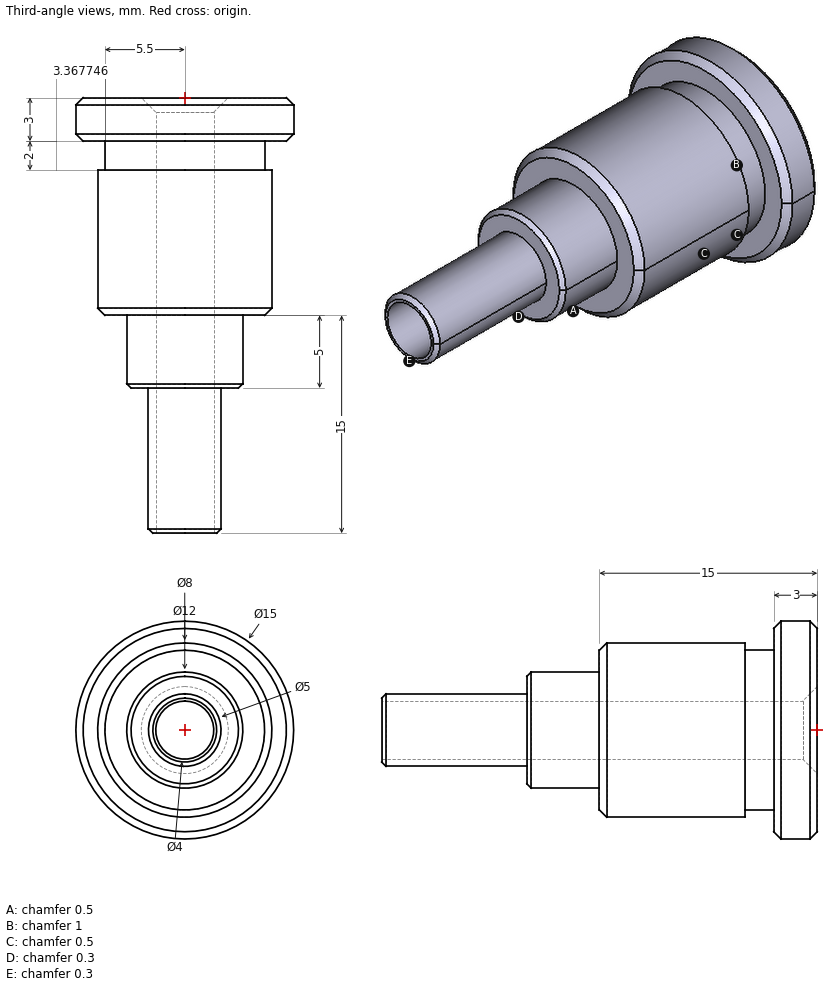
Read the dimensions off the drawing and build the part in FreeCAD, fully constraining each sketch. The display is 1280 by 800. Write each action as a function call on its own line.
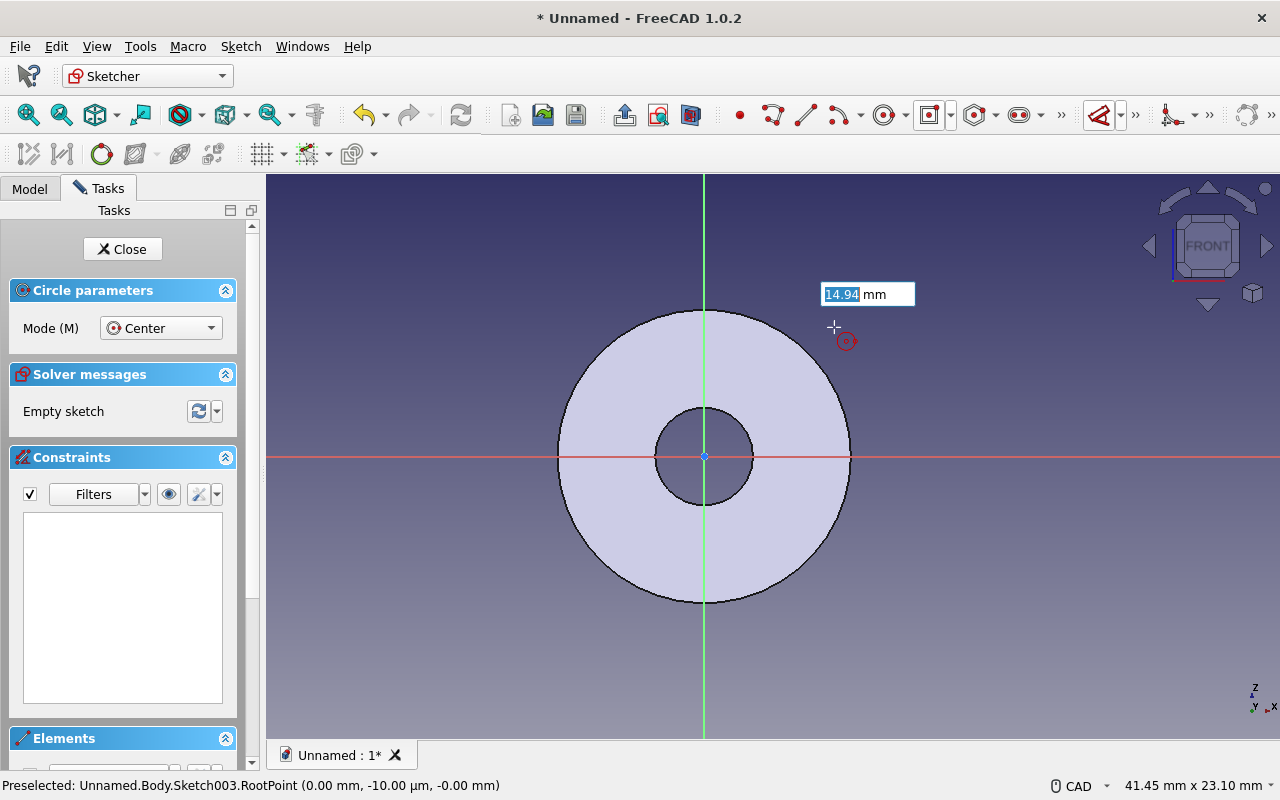
text(15)
key(Return)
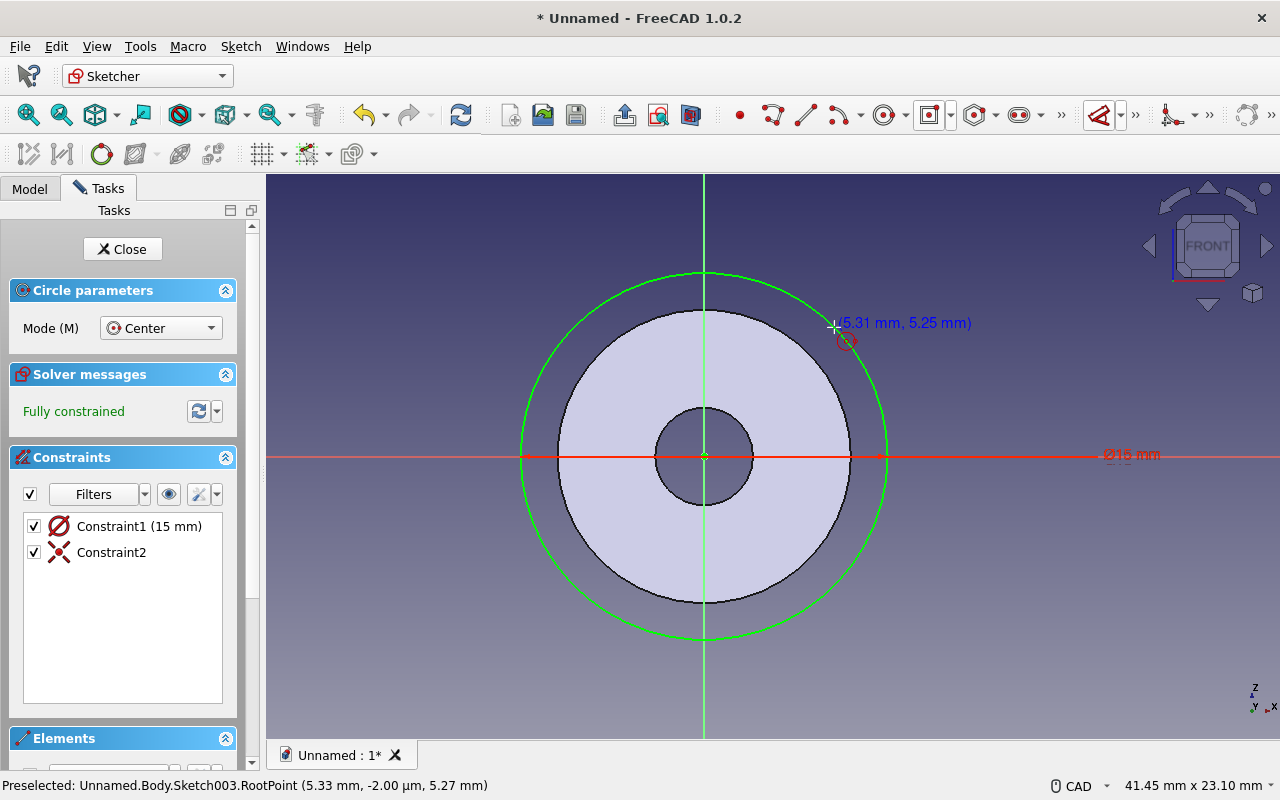
click(704, 456)
move(808, 353)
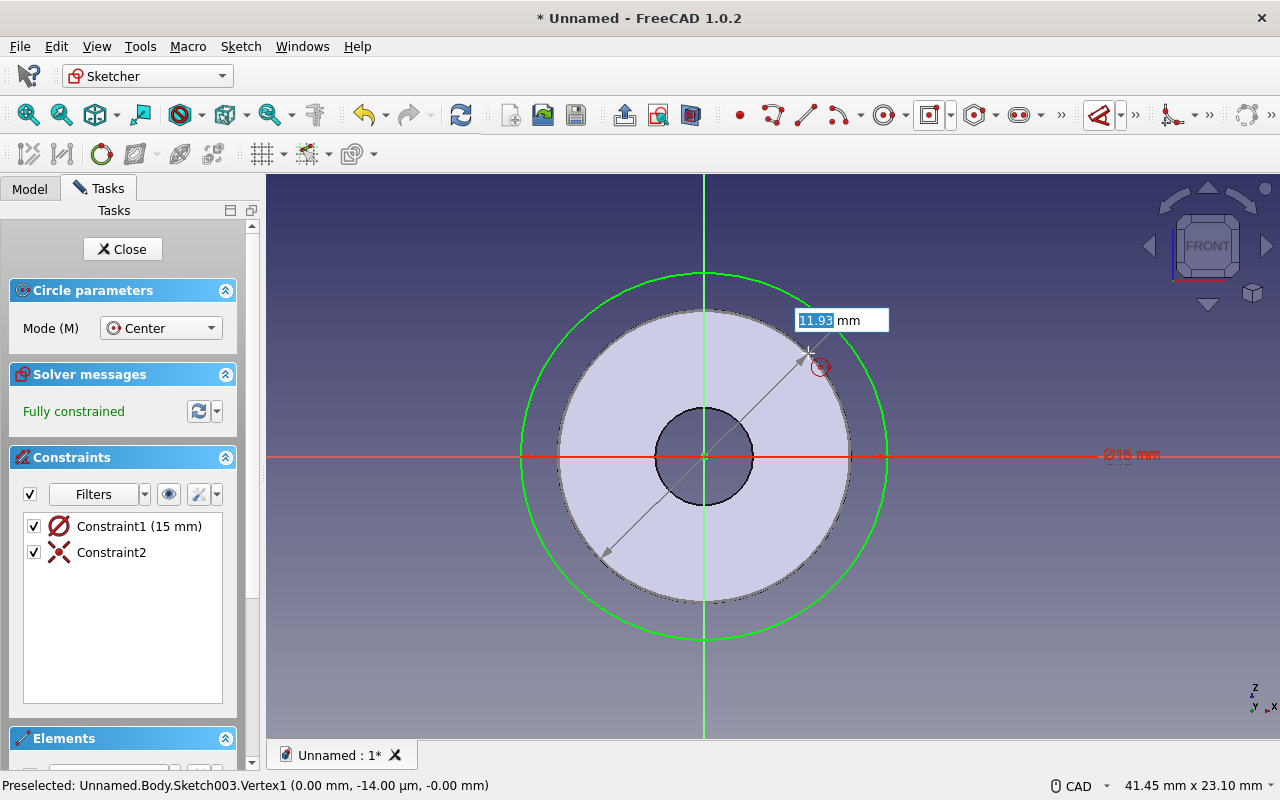
text(12)
key(Return)
key(Escape)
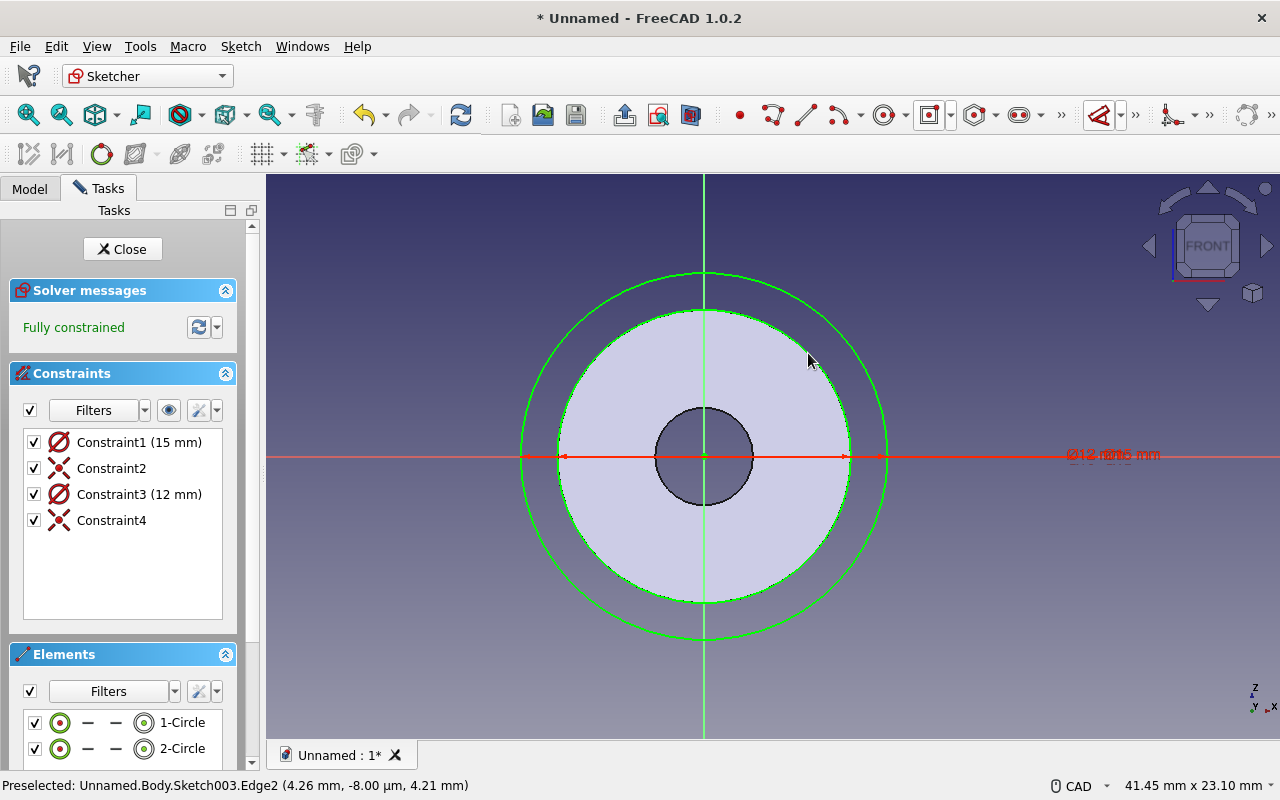
click(123, 249)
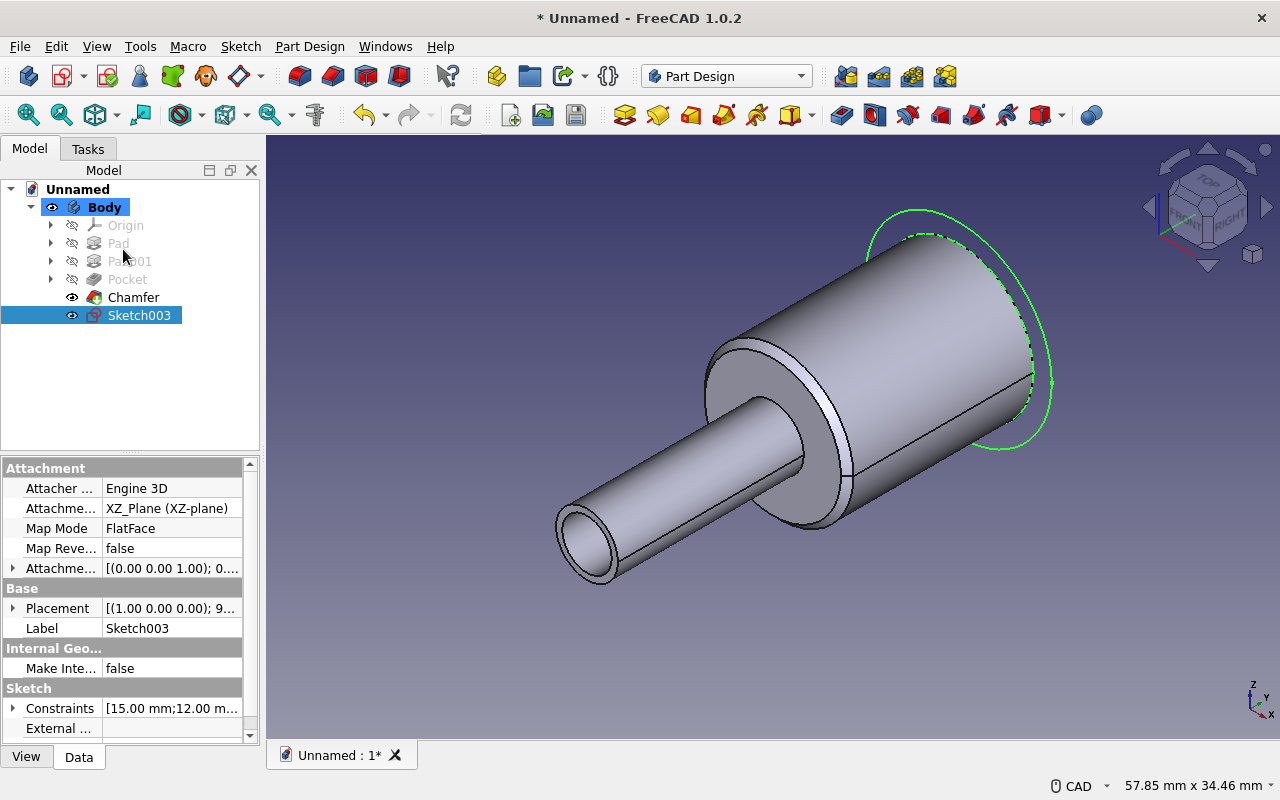
click(625, 116)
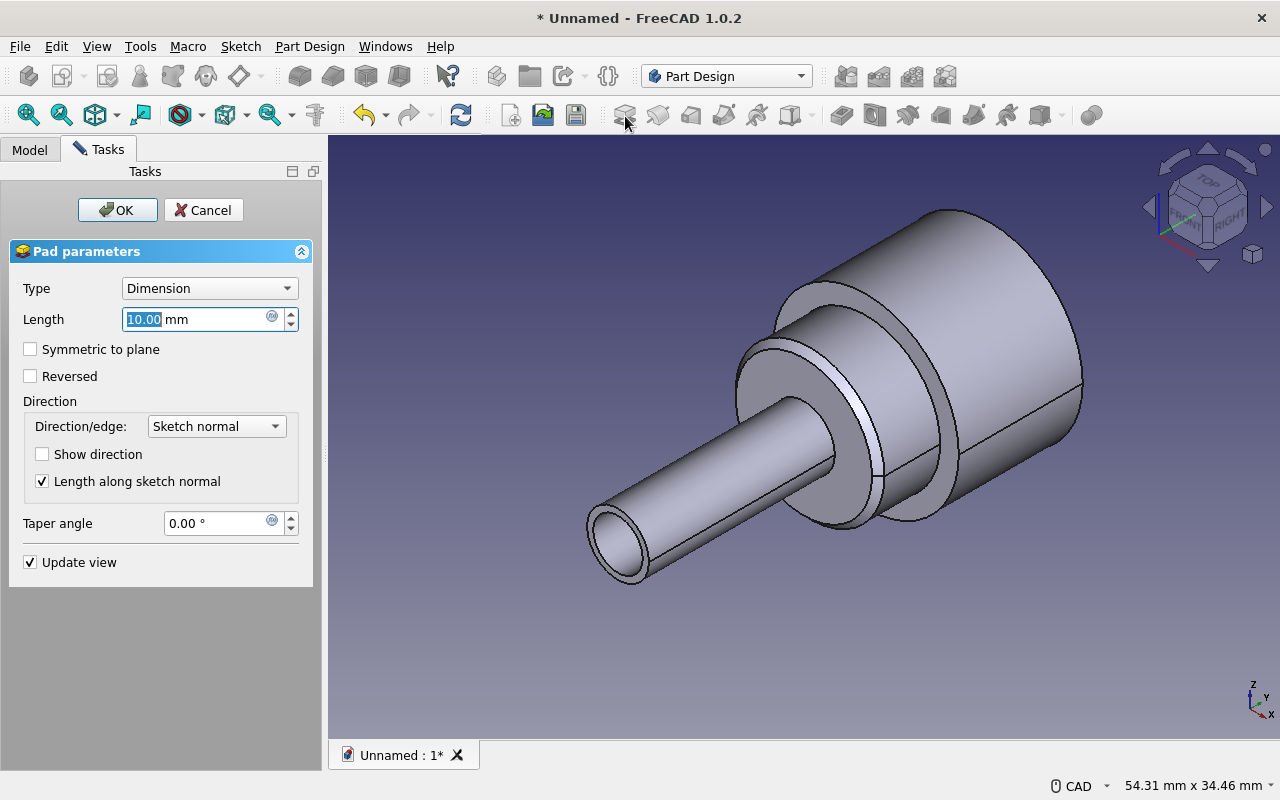
text(3)
key(Tab)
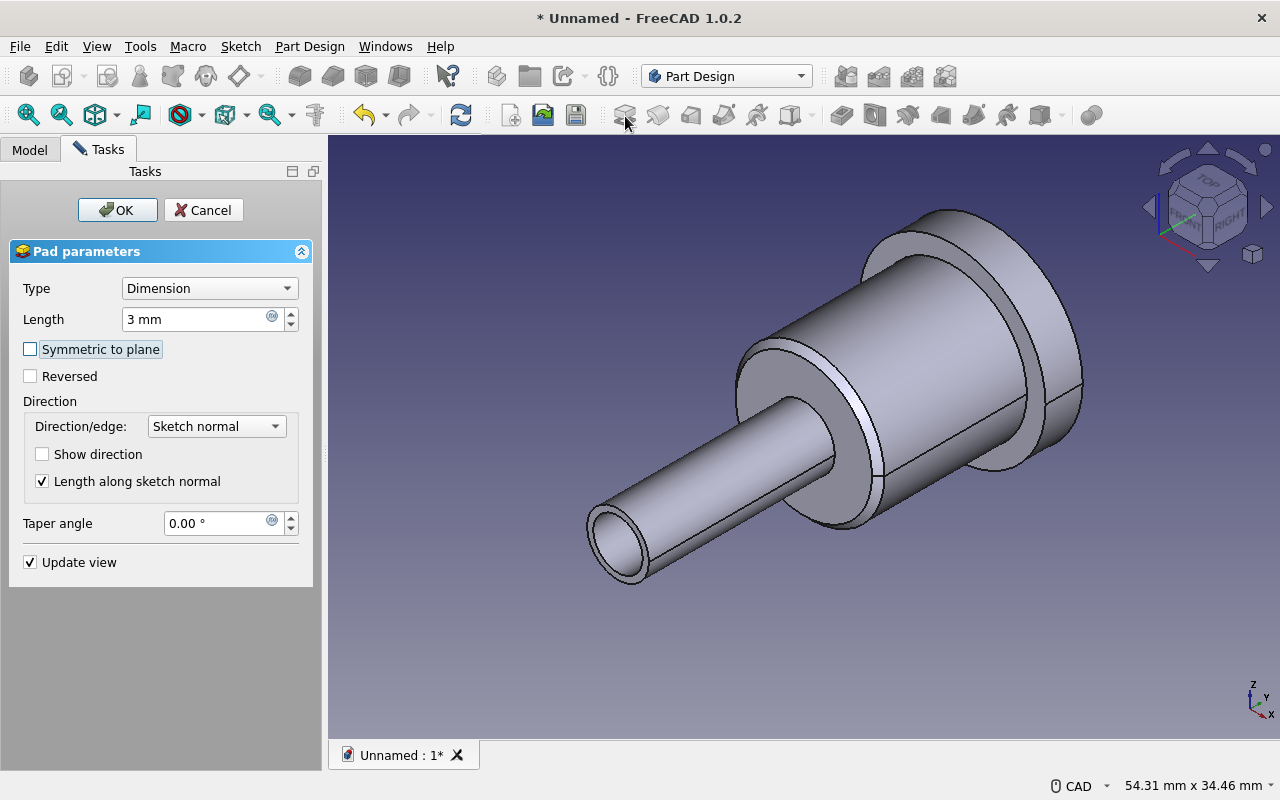
click(118, 210)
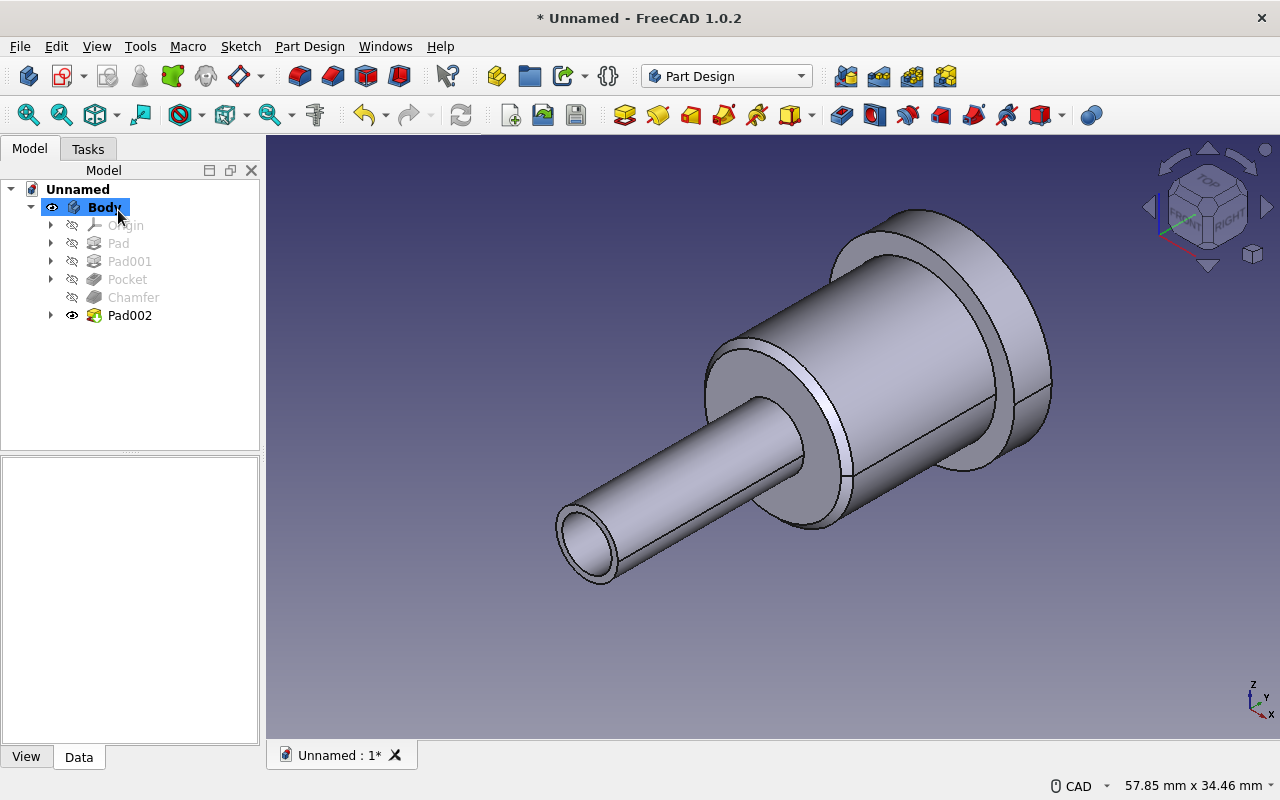
key(2)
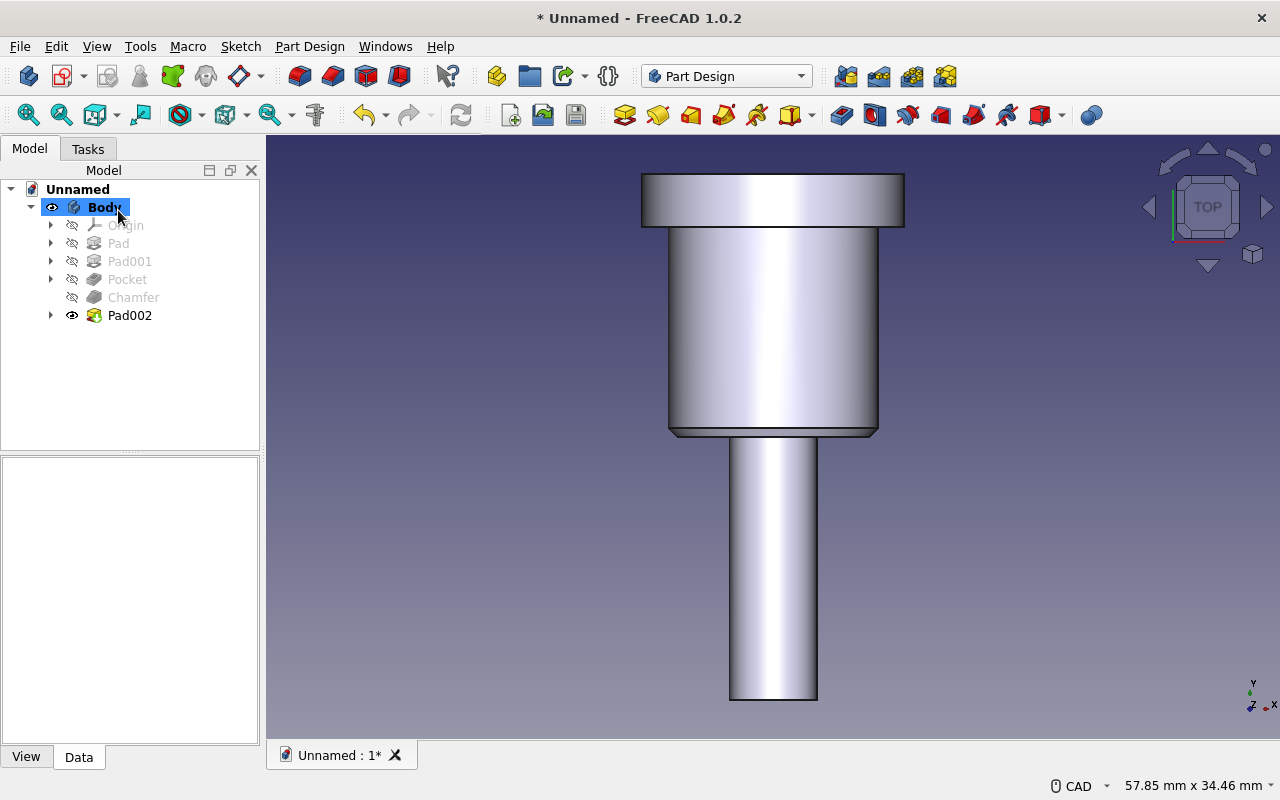
key(0)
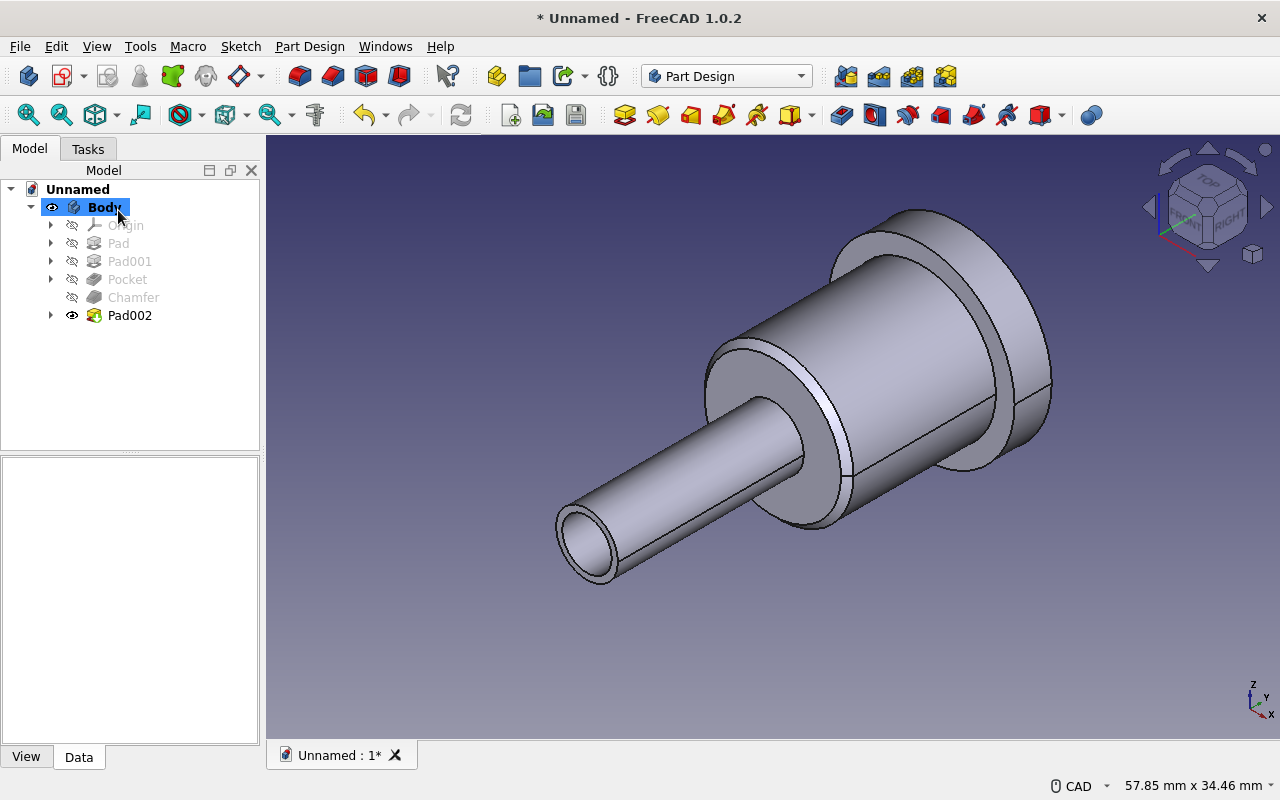
key(1)